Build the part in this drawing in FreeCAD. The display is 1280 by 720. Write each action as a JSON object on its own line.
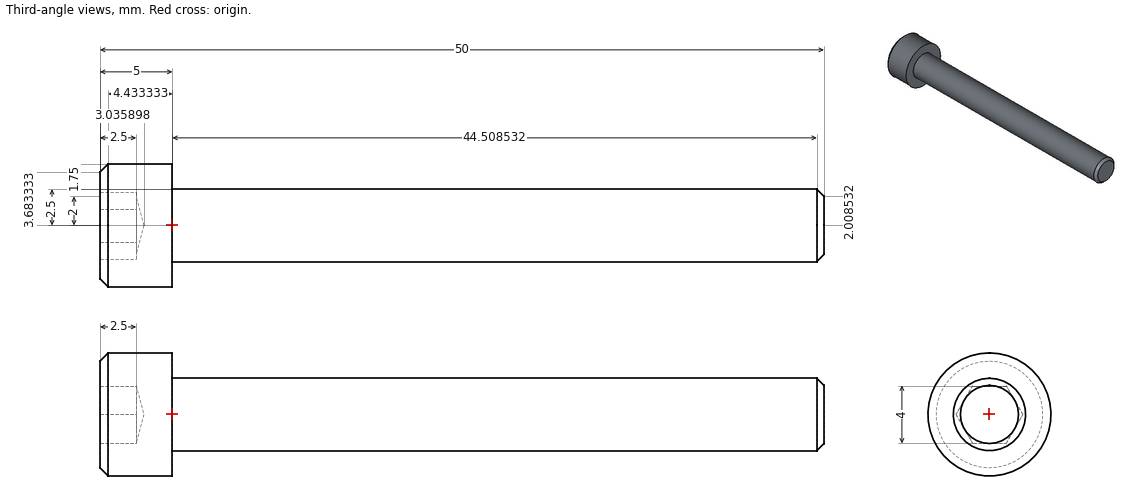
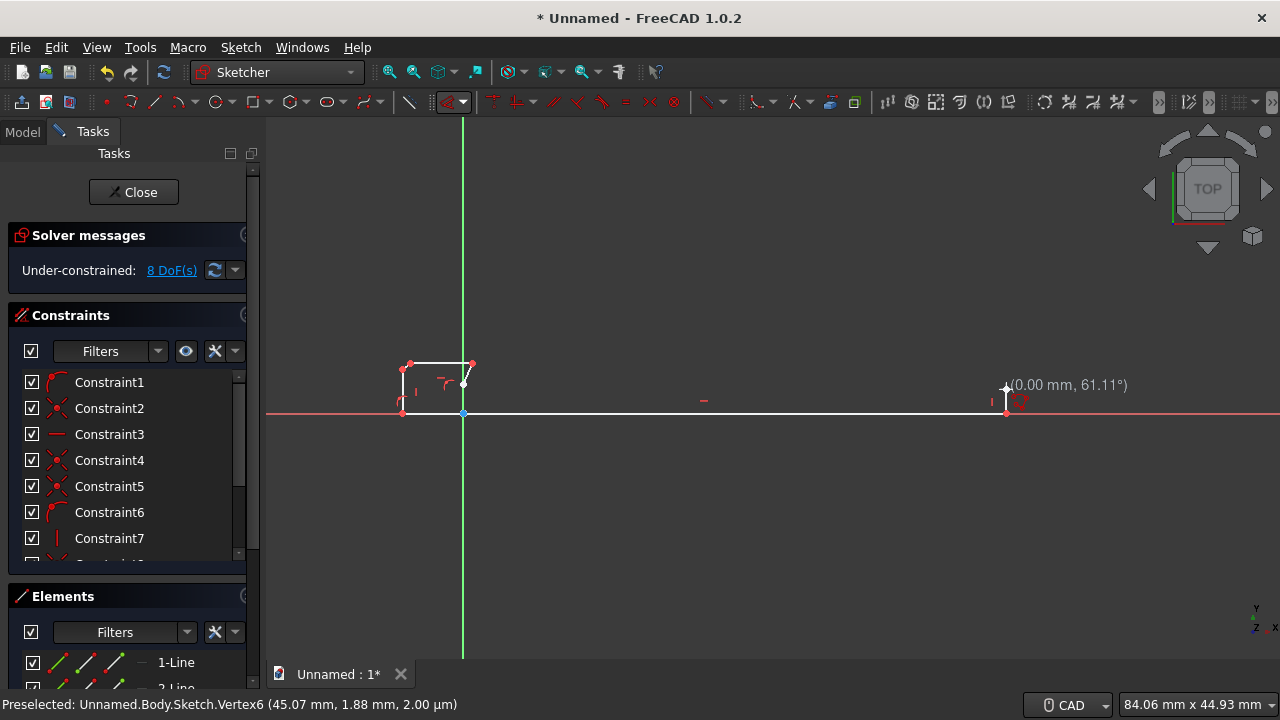
{"action": "scroll", "coordinate": [1000, 383], "scroll_direction": "up", "scroll_amount": 4}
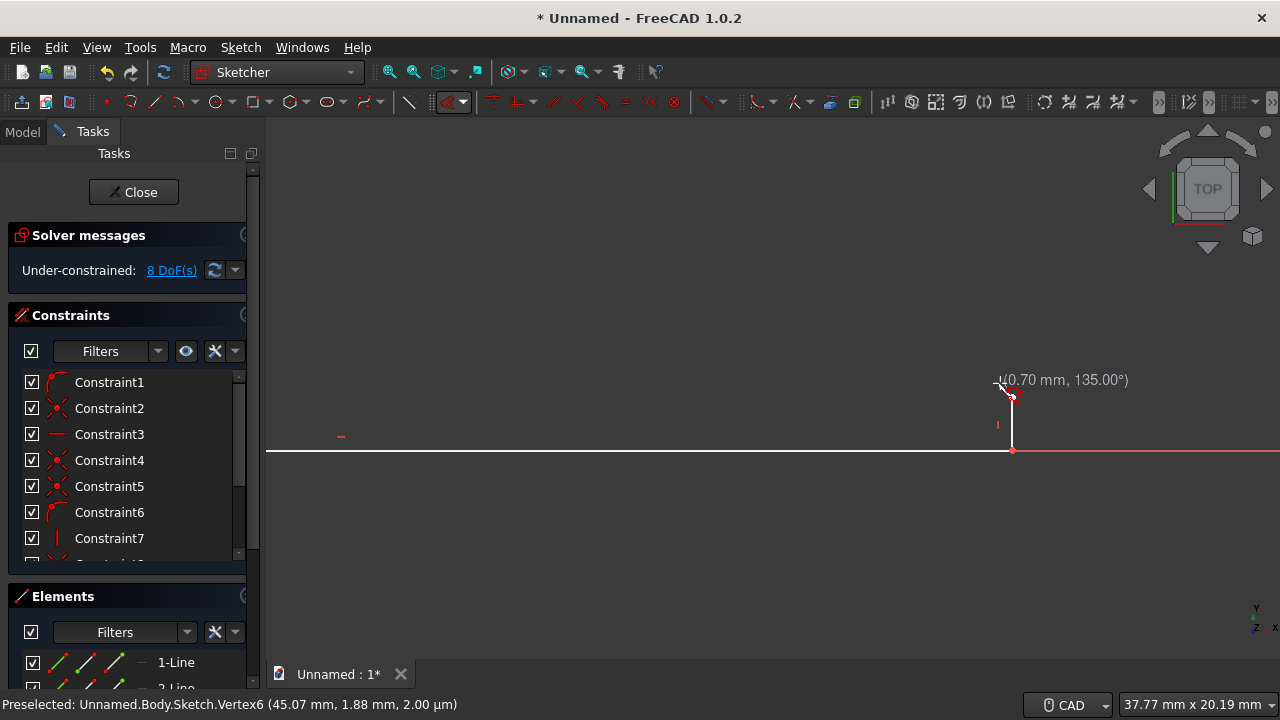
{"action": "left_click", "coordinate": [1000, 383]}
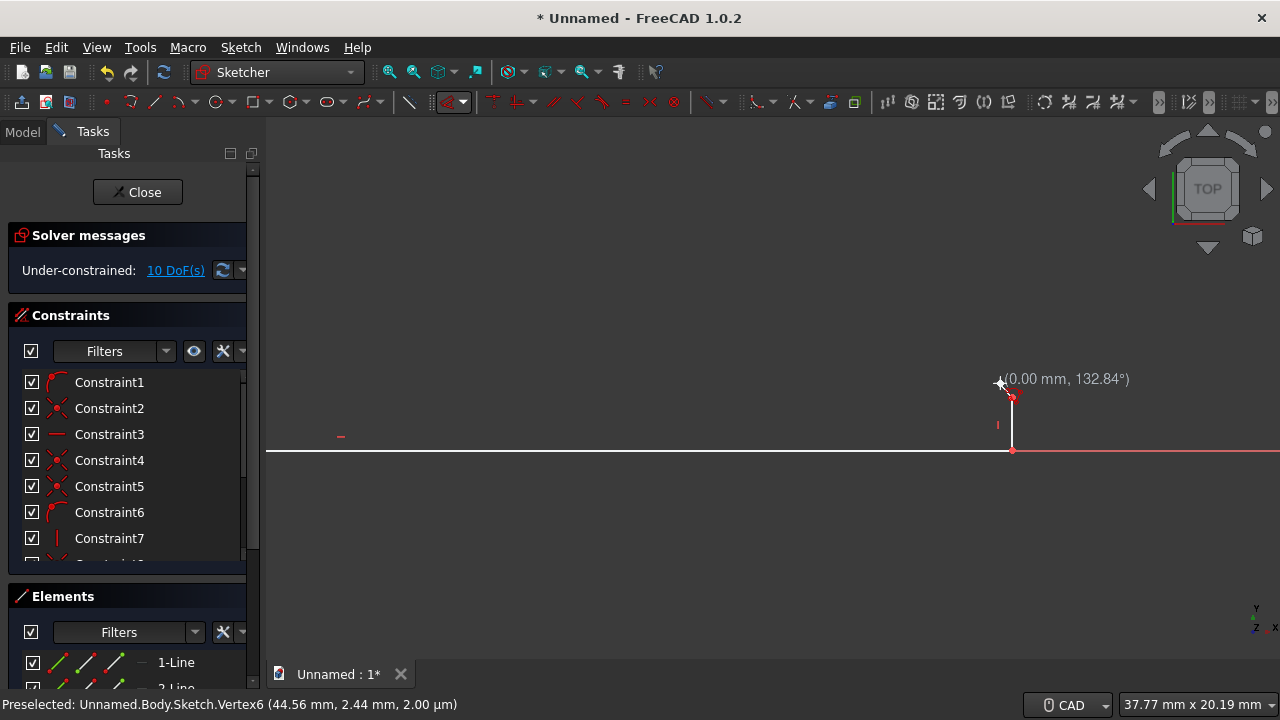
{"action": "scroll", "coordinate": [1001, 384], "scroll_direction": "down", "scroll_amount": 4}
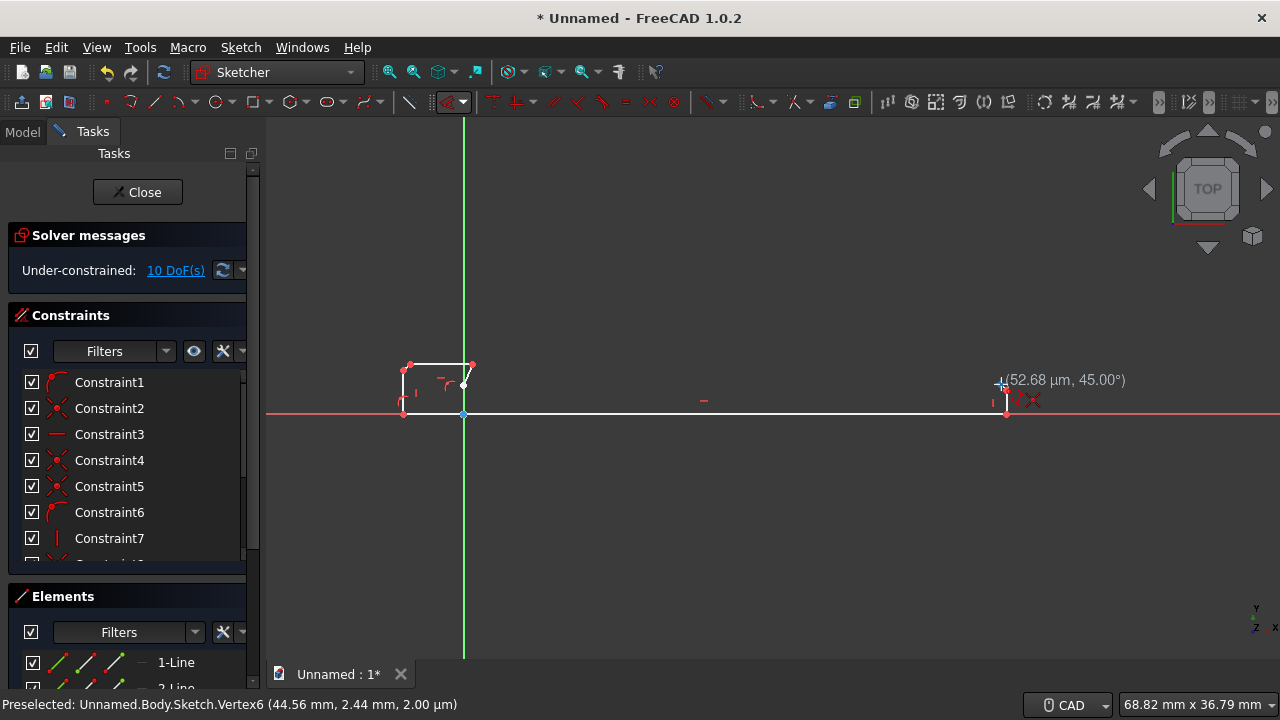
{"action": "scroll", "coordinate": [464, 384], "scroll_direction": "up", "scroll_amount": 3}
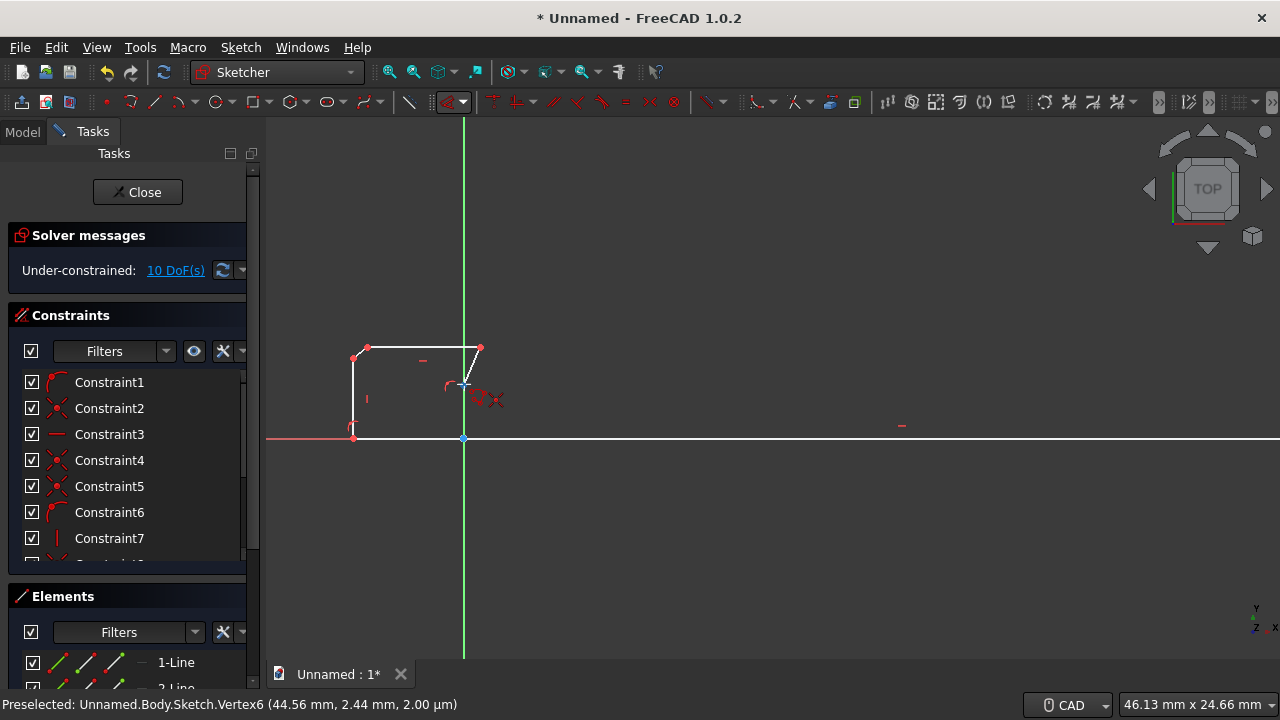
{"action": "left_click", "coordinate": [464, 385]}
{"action": "key", "text": "Escape"}
{"action": "key", "text": "Escape"}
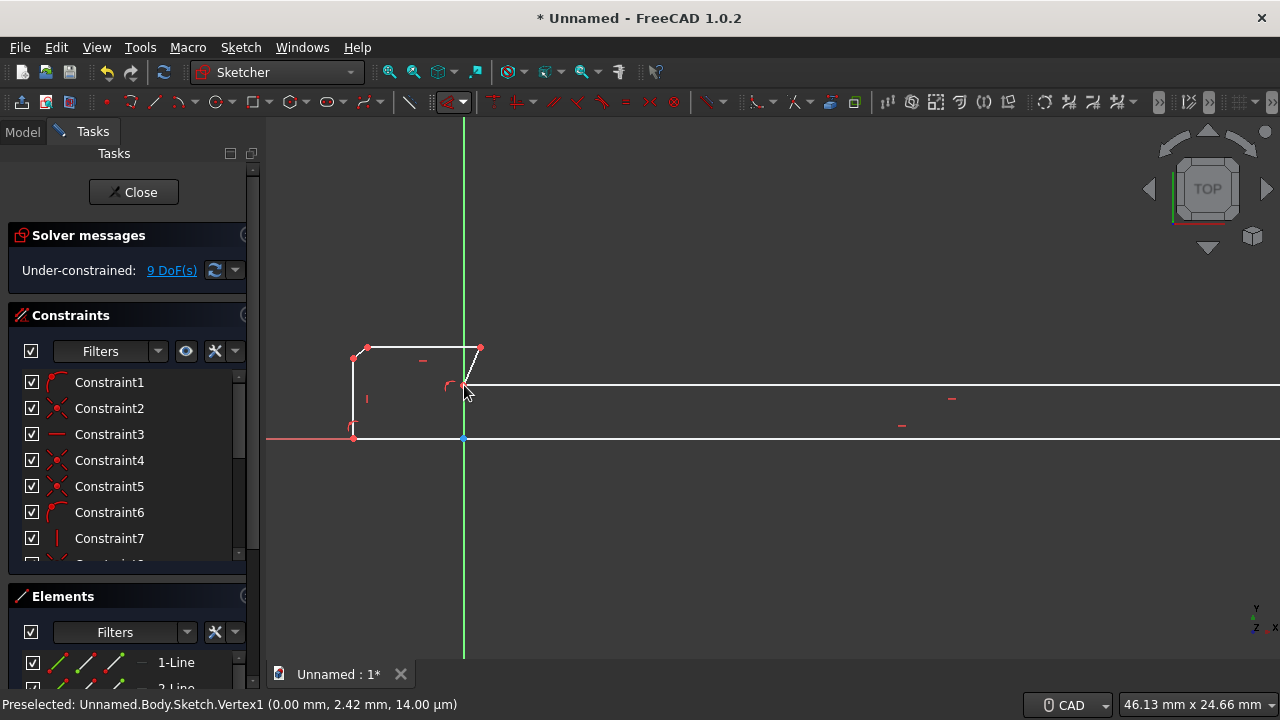
{"action": "left_click", "coordinate": [475, 359]}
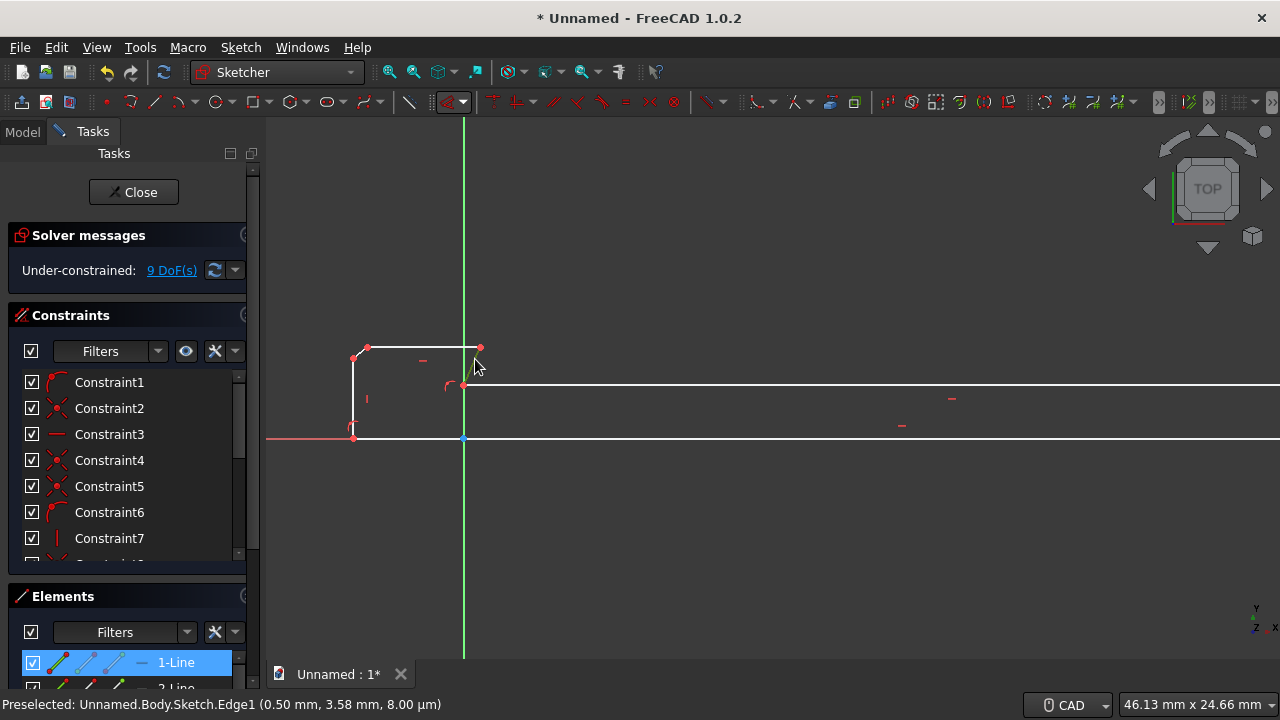
{"action": "key", "text": "v"}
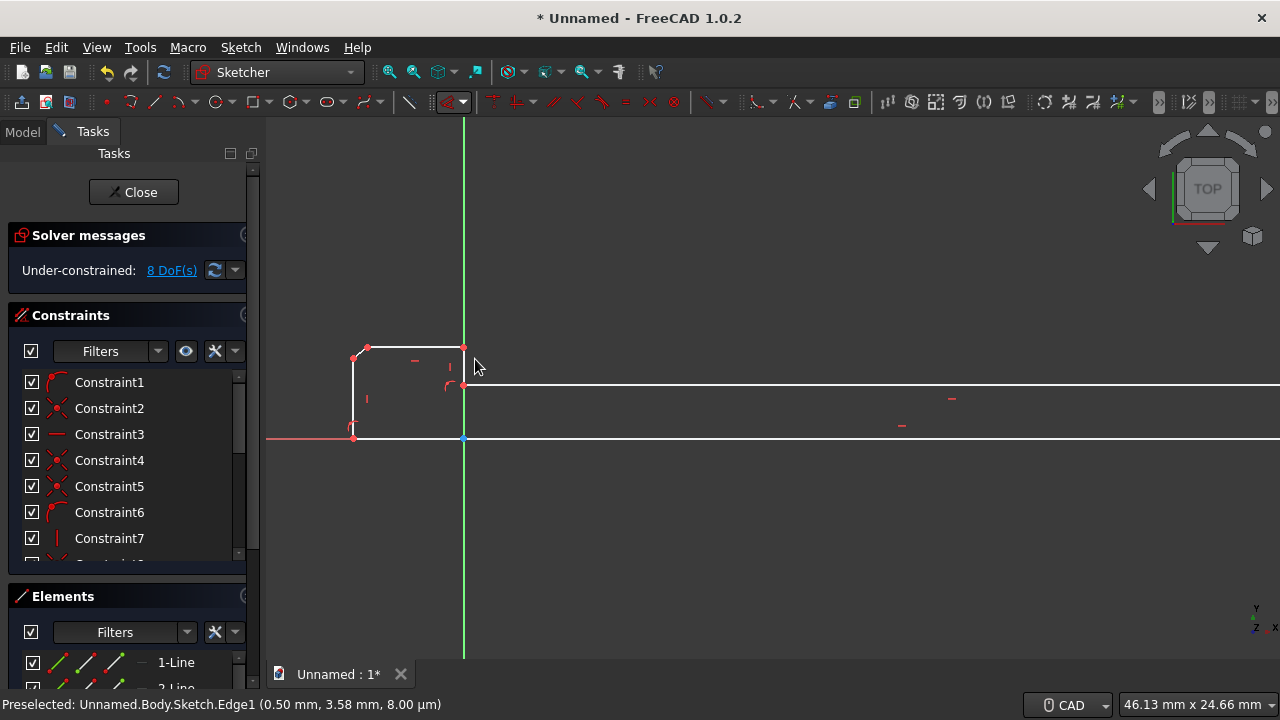
{"action": "left_click", "coordinate": [448, 102]}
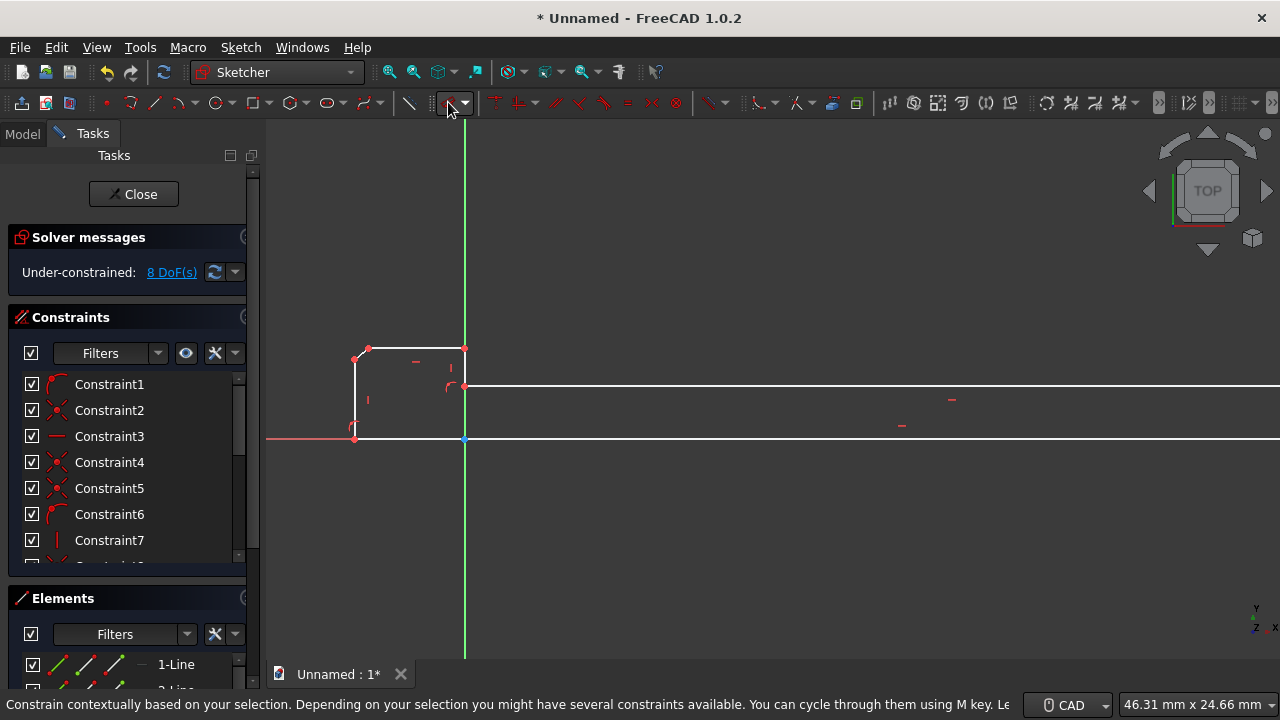
{"action": "left_click", "coordinate": [683, 439]}
{"action": "left_click", "coordinate": [735, 473]}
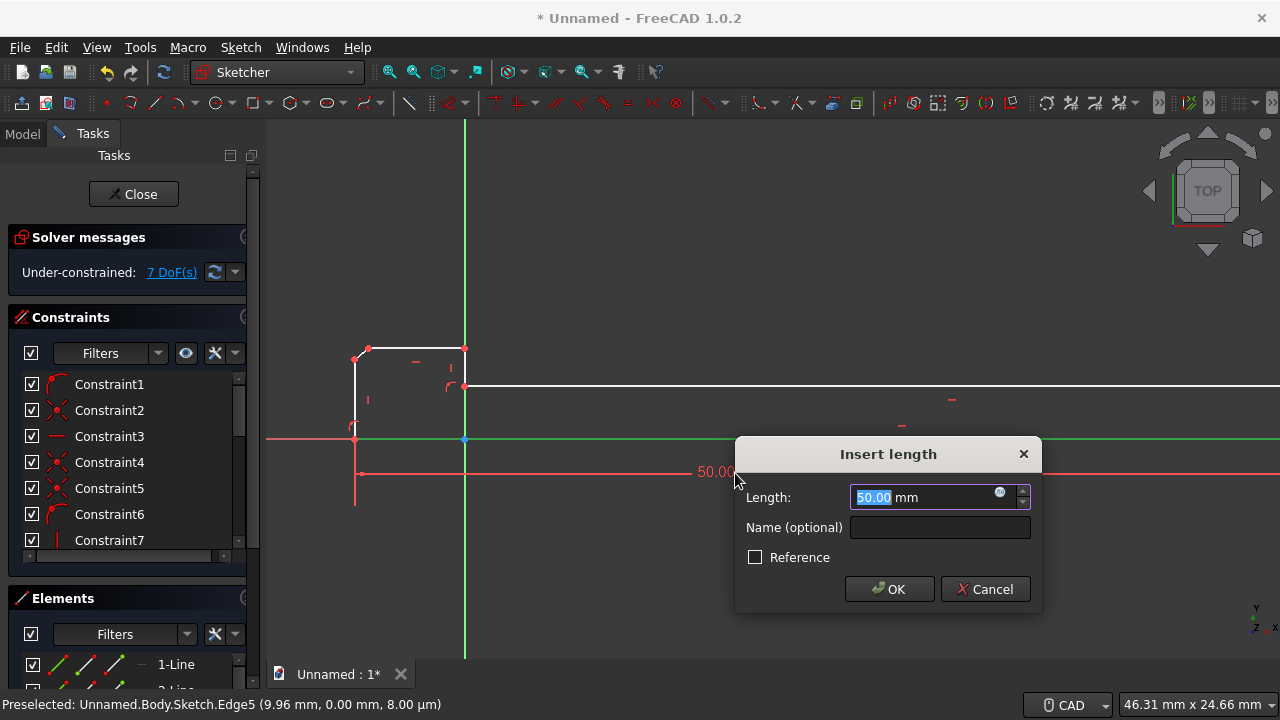
{"action": "type", "text": "50"}
{"action": "key", "text": "Return"}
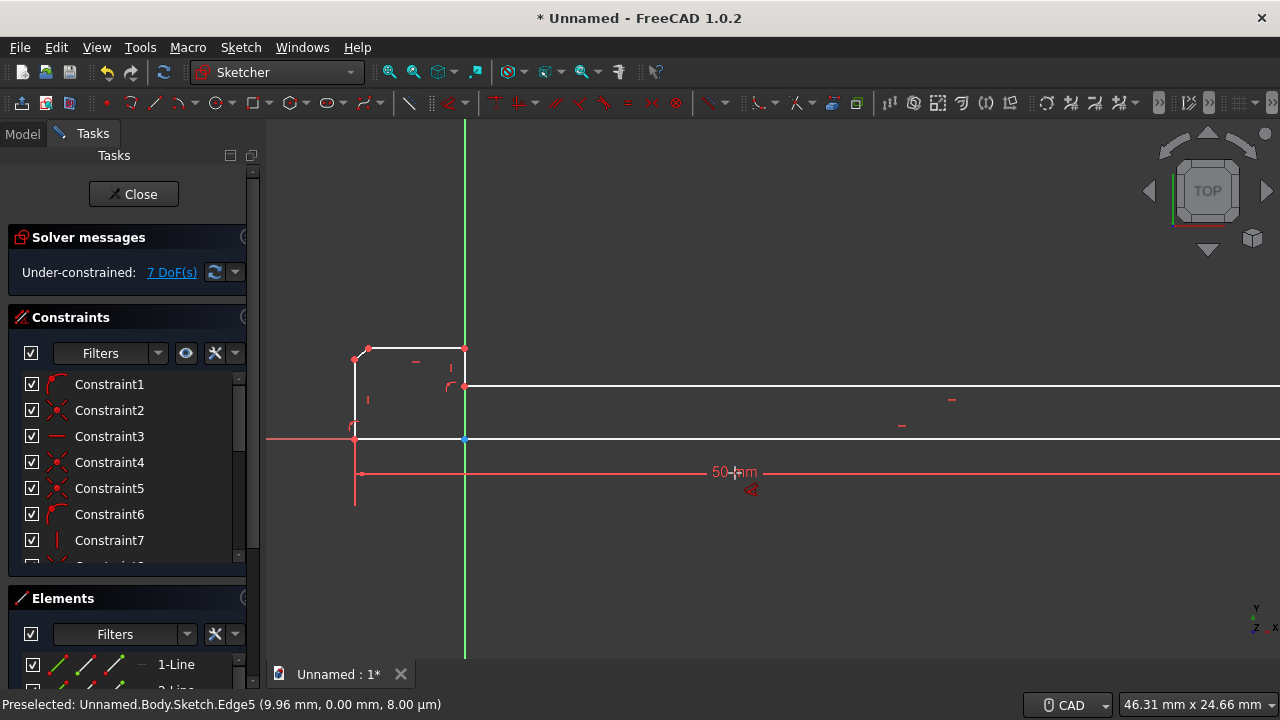
{"action": "left_click", "coordinate": [355, 360]}
{"action": "left_click", "coordinate": [410, 473]}